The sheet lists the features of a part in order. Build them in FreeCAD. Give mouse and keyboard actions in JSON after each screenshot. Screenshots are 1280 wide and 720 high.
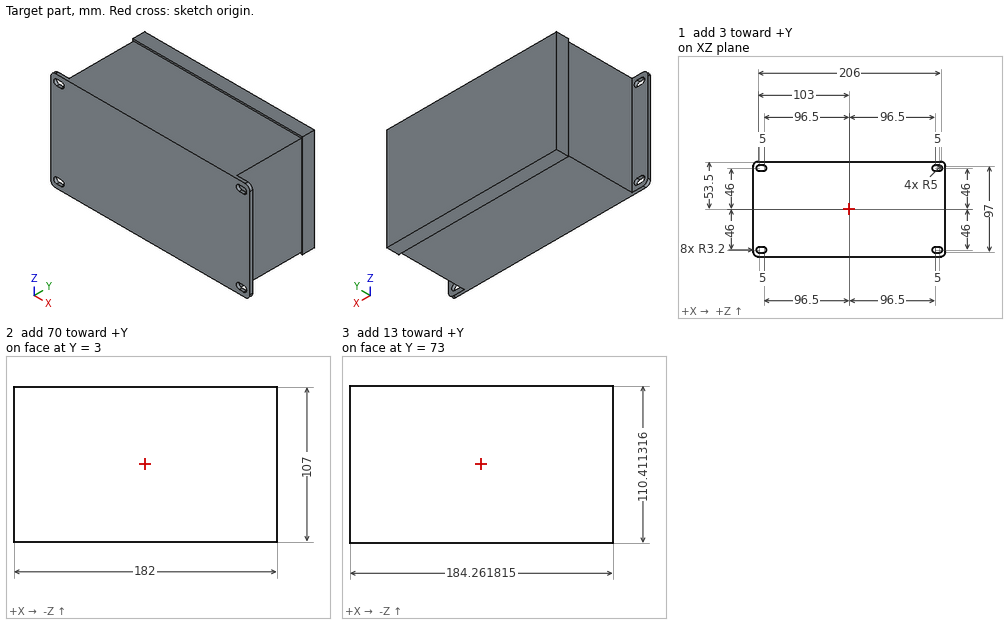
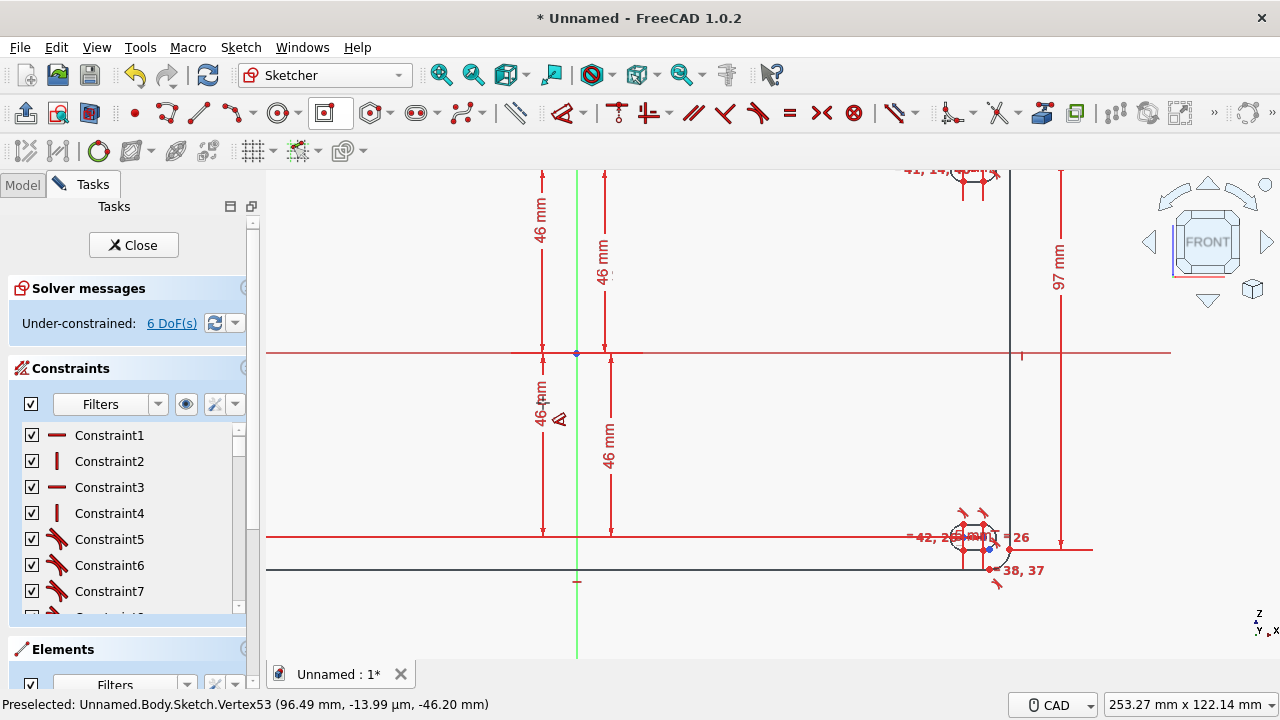
{"action": "scroll", "coordinate": [964, 539], "scroll_direction": "down", "scroll_amount": 2}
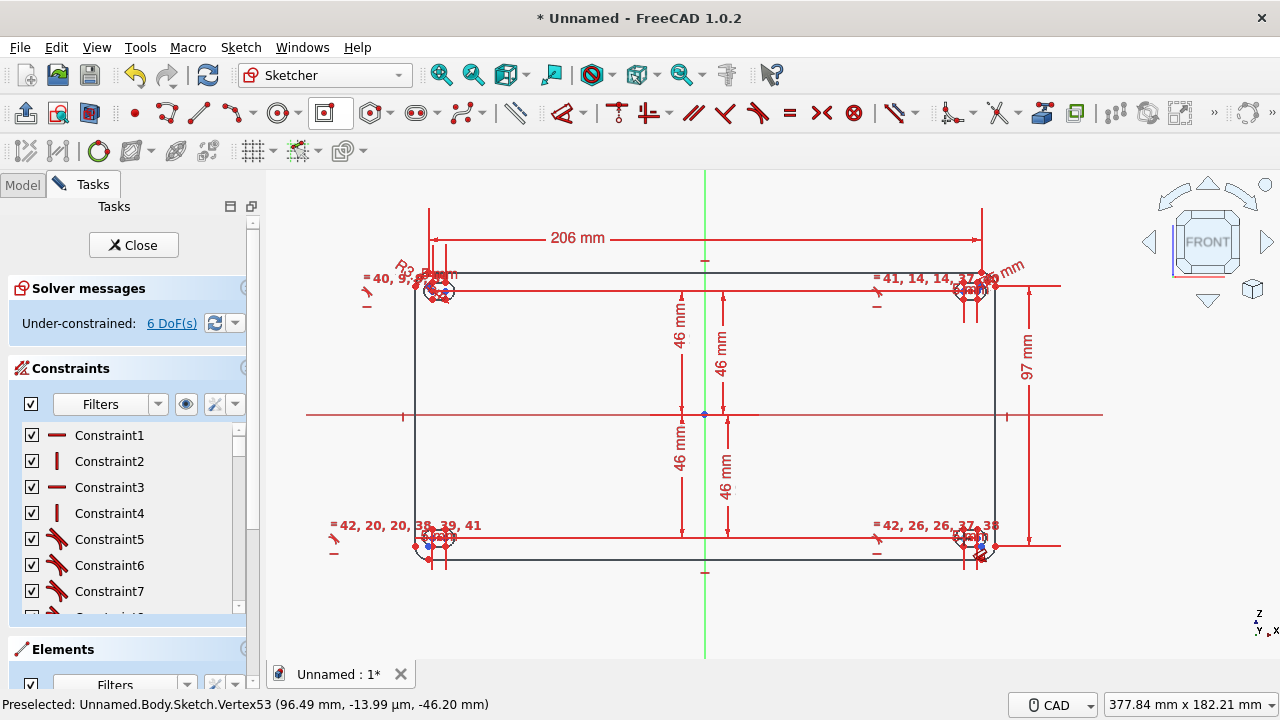
{"action": "left_click", "coordinate": [429, 273]}
{"action": "left_click", "coordinate": [503, 239]}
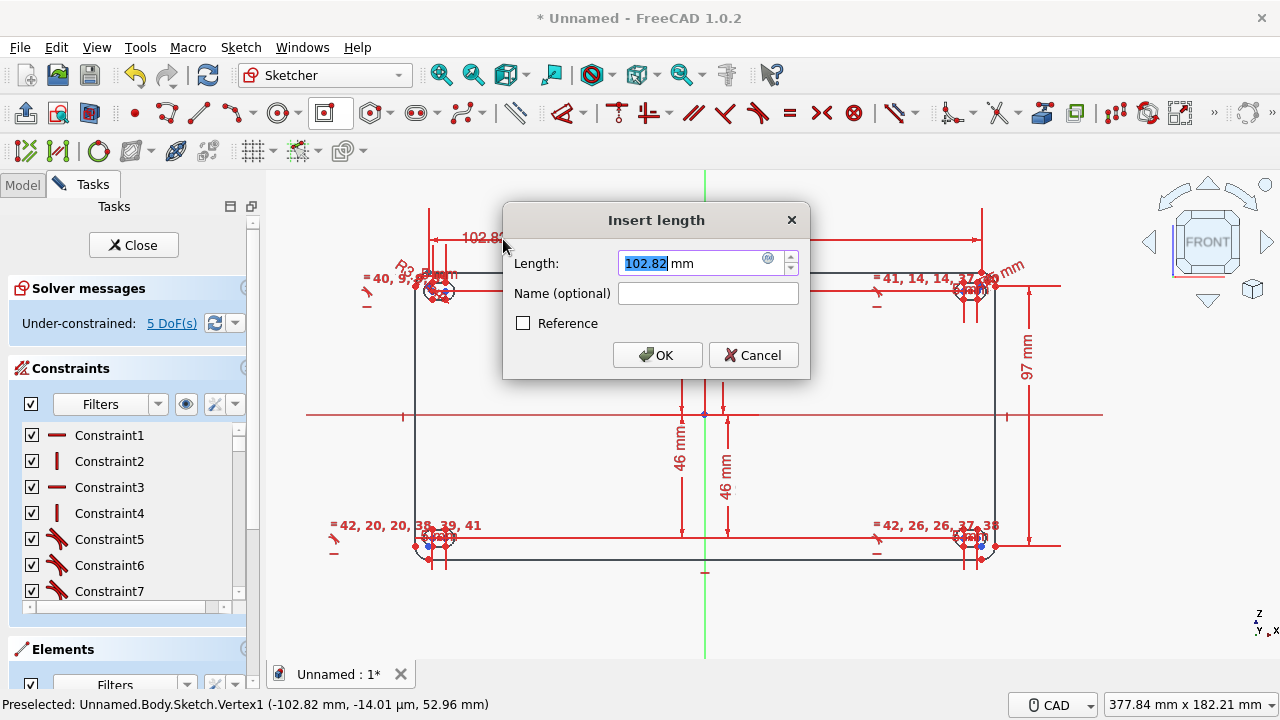
{"action": "type", "text": "103"}
{"action": "key", "text": "Return"}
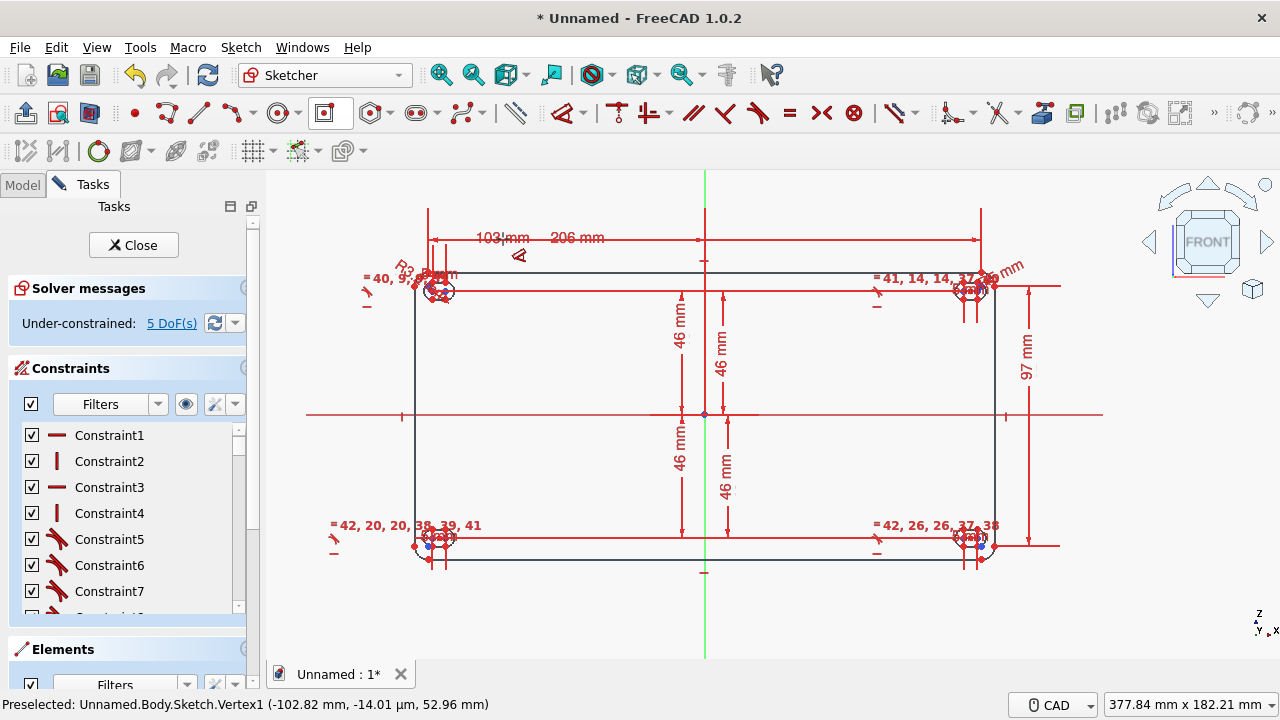
{"action": "left_click", "coordinate": [428, 273]}
{"action": "left_click", "coordinate": [394, 344]}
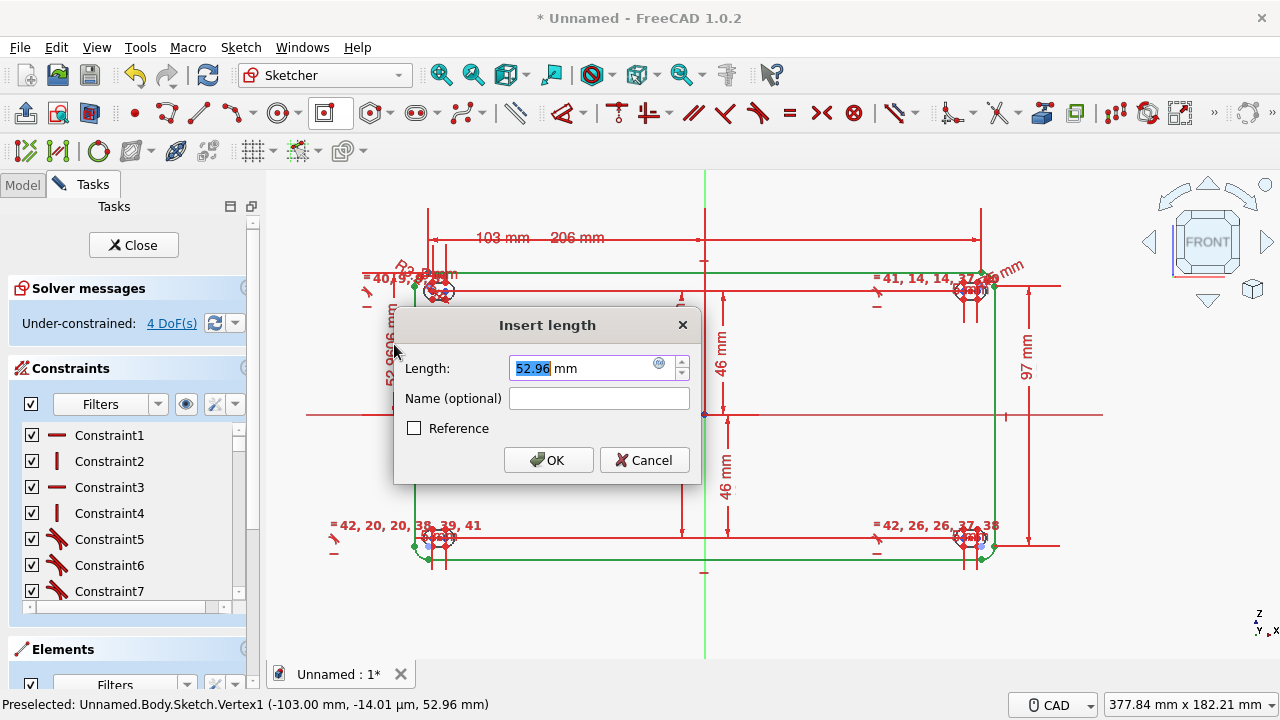
{"action": "type", "text": "53.5"}
{"action": "key", "text": "Return"}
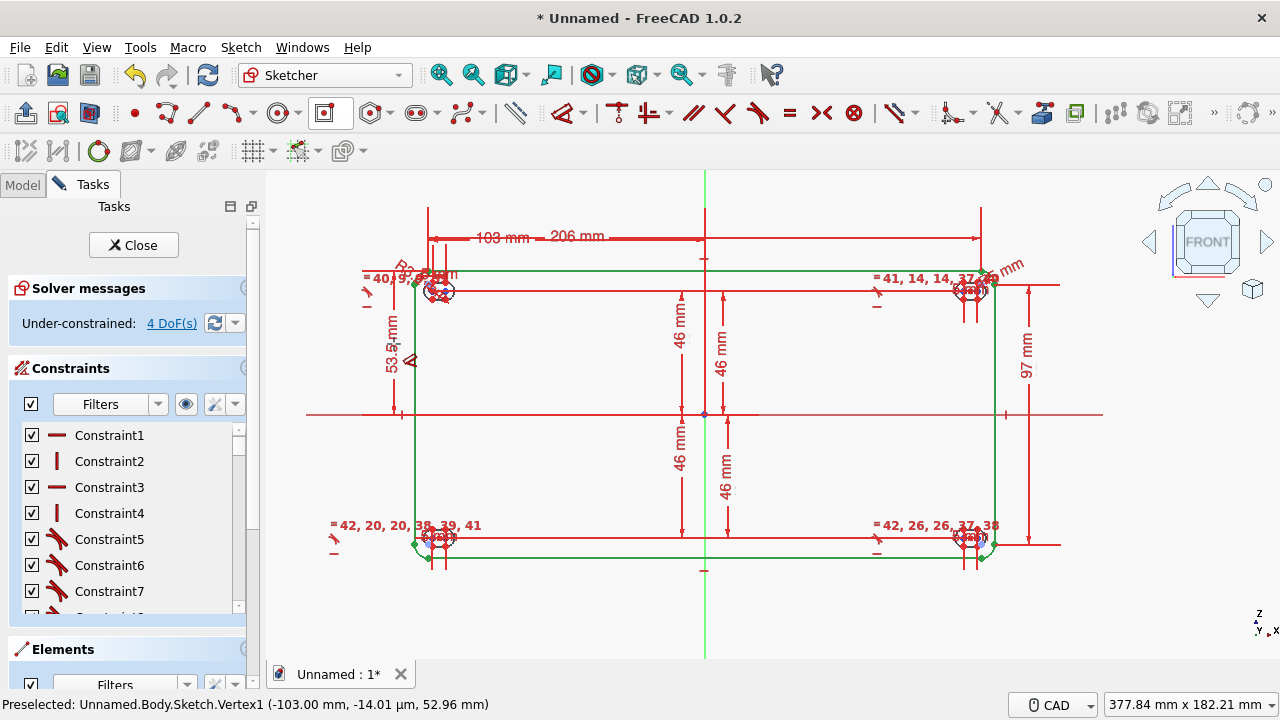
{"action": "scroll", "coordinate": [446, 300], "scroll_direction": "up", "scroll_amount": 2}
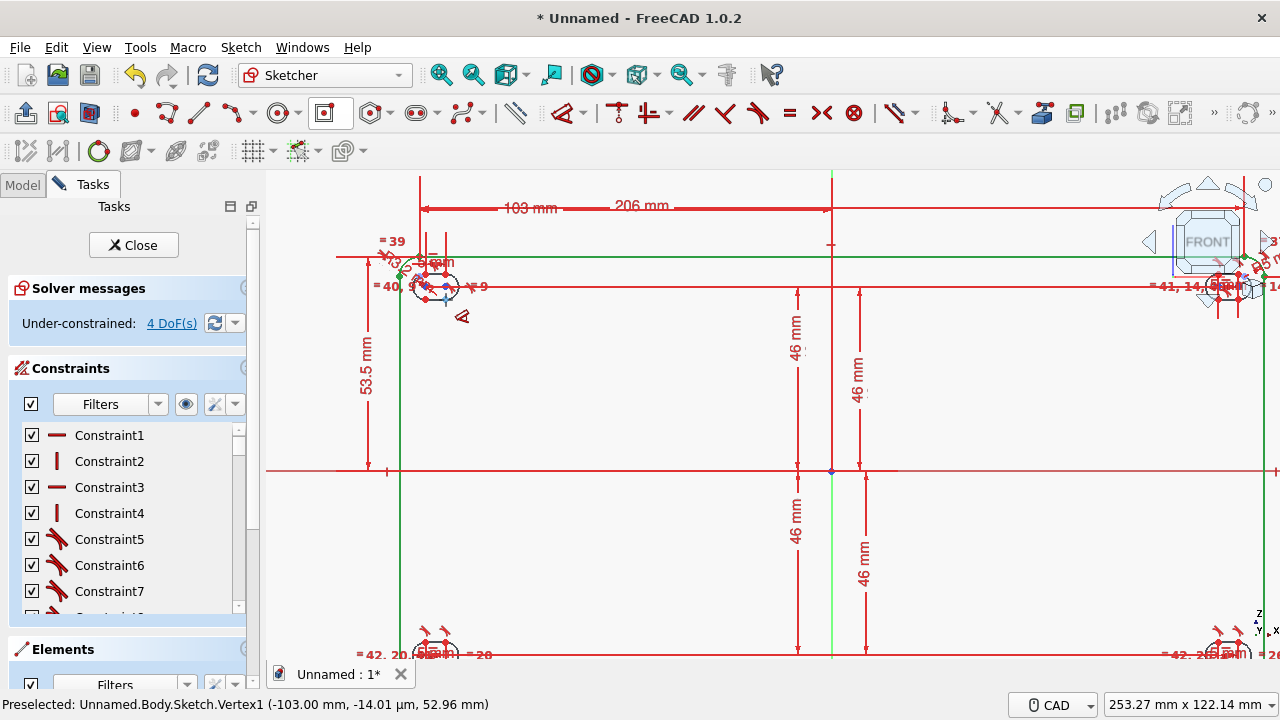
{"action": "left_click", "coordinate": [446, 300]}
{"action": "left_click", "coordinate": [639, 505]}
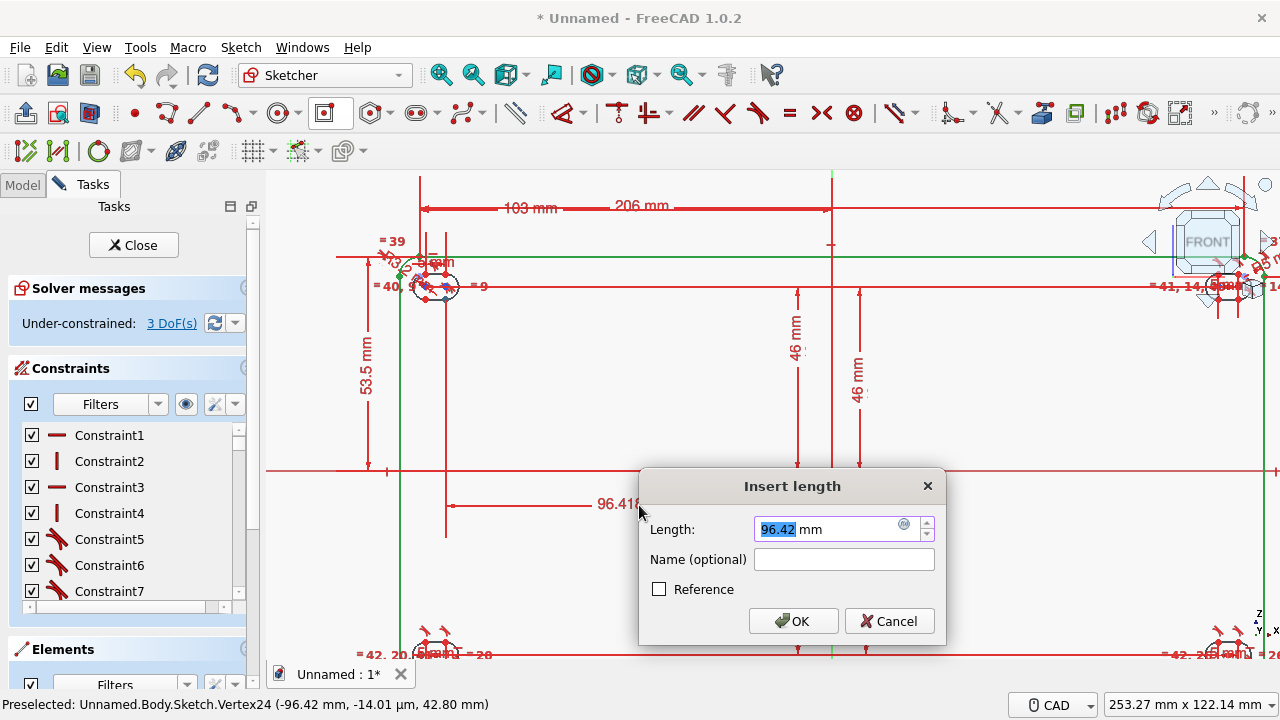
{"action": "type", "text": "96.5"}
{"action": "key", "text": "Return"}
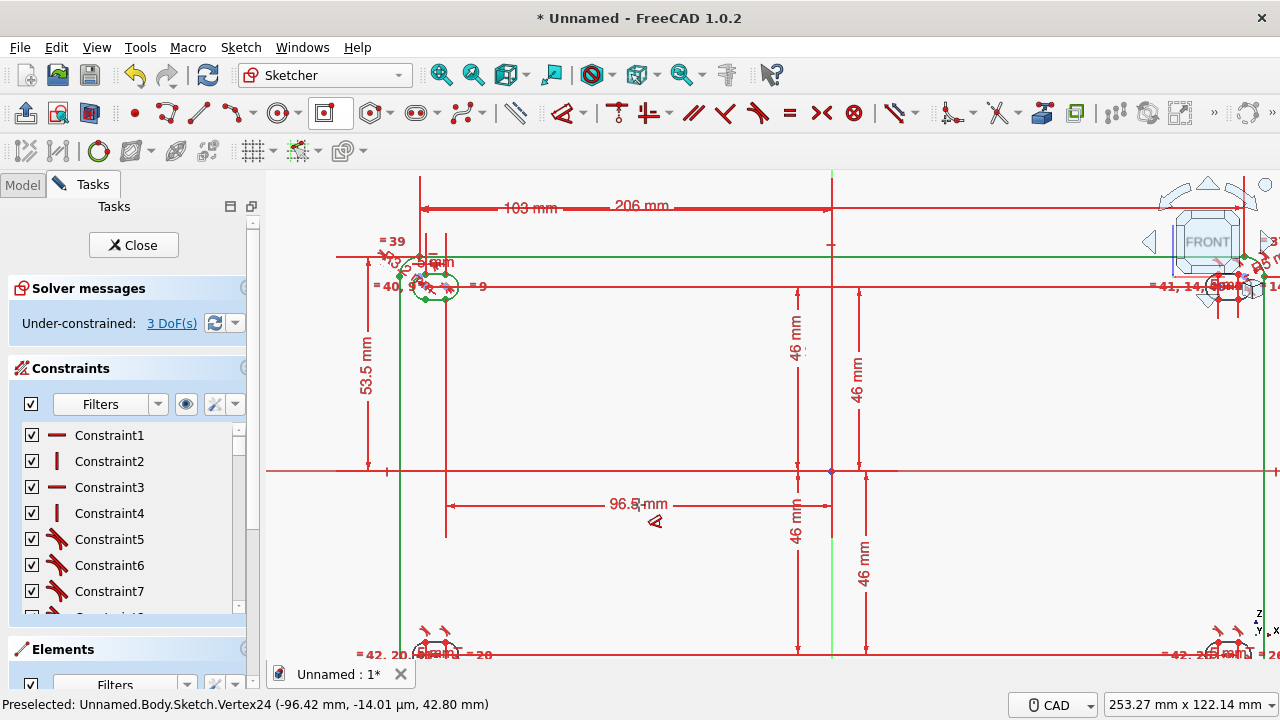
{"action": "scroll", "coordinate": [445, 299], "scroll_direction": "down", "scroll_amount": 2}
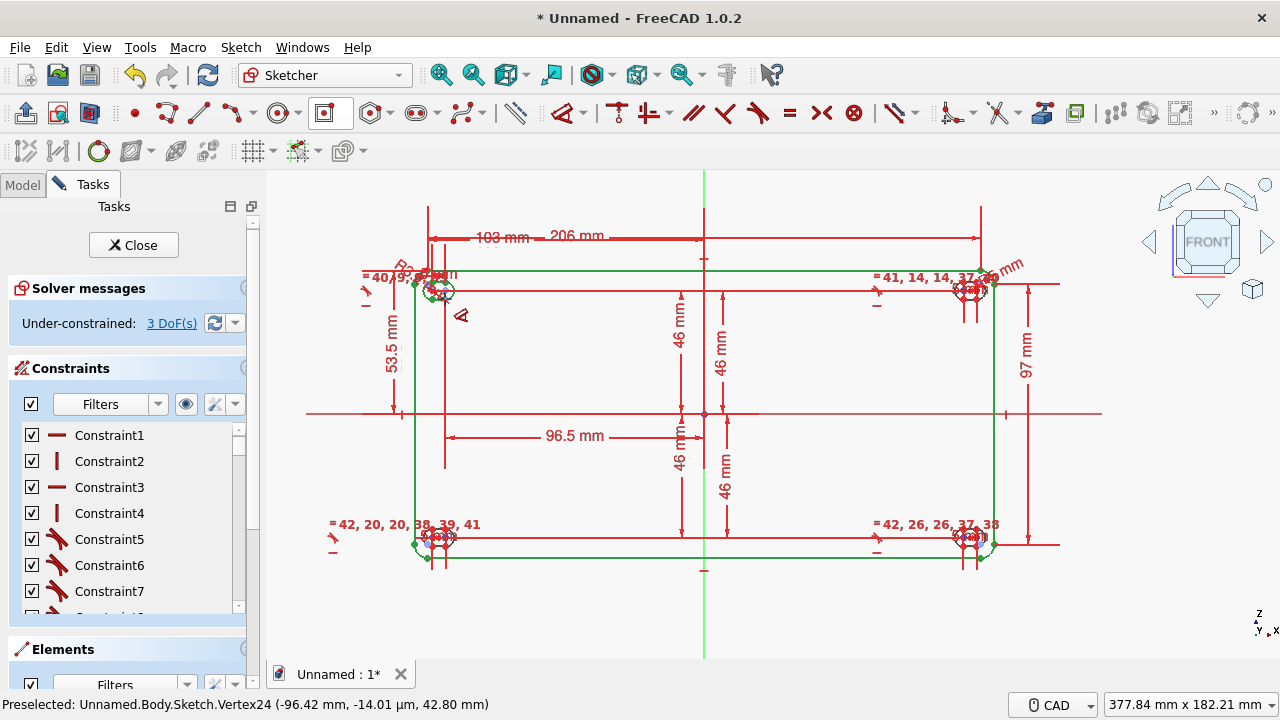
{"action": "scroll", "coordinate": [964, 282], "scroll_direction": "up", "scroll_amount": 2}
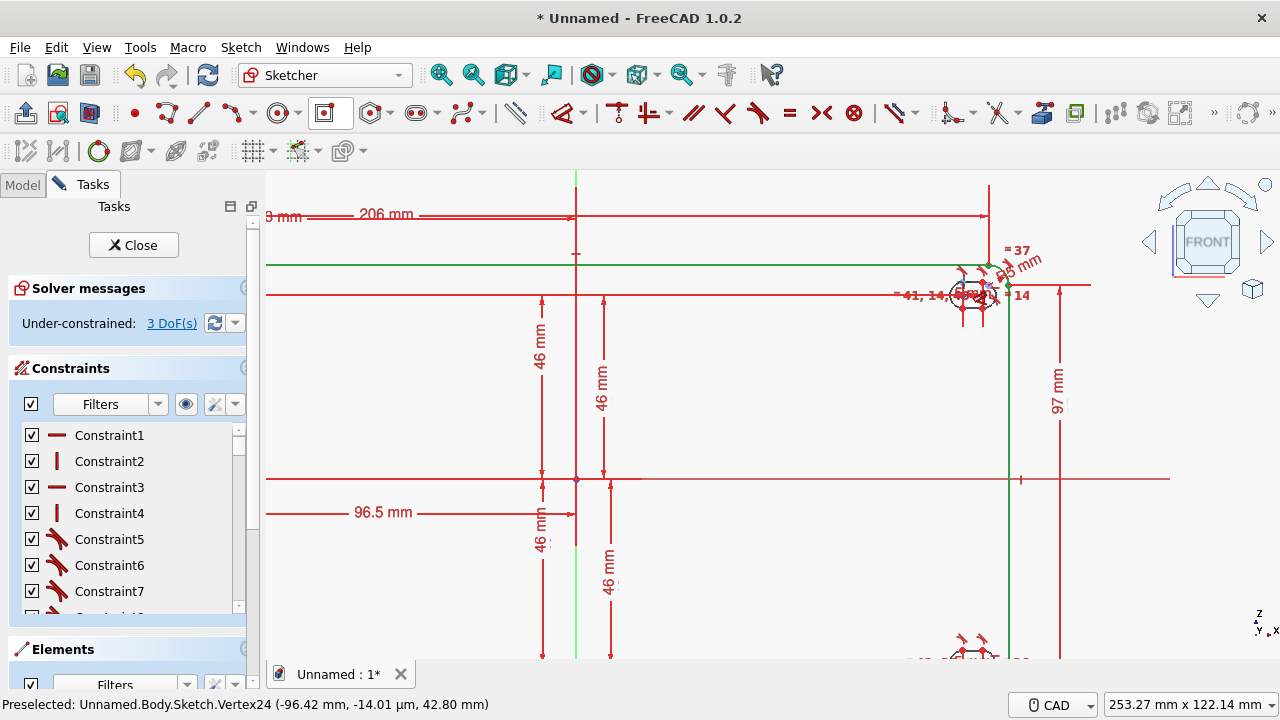
{"action": "left_click", "coordinate": [963, 282]}
{"action": "left_click", "coordinate": [770, 248]}